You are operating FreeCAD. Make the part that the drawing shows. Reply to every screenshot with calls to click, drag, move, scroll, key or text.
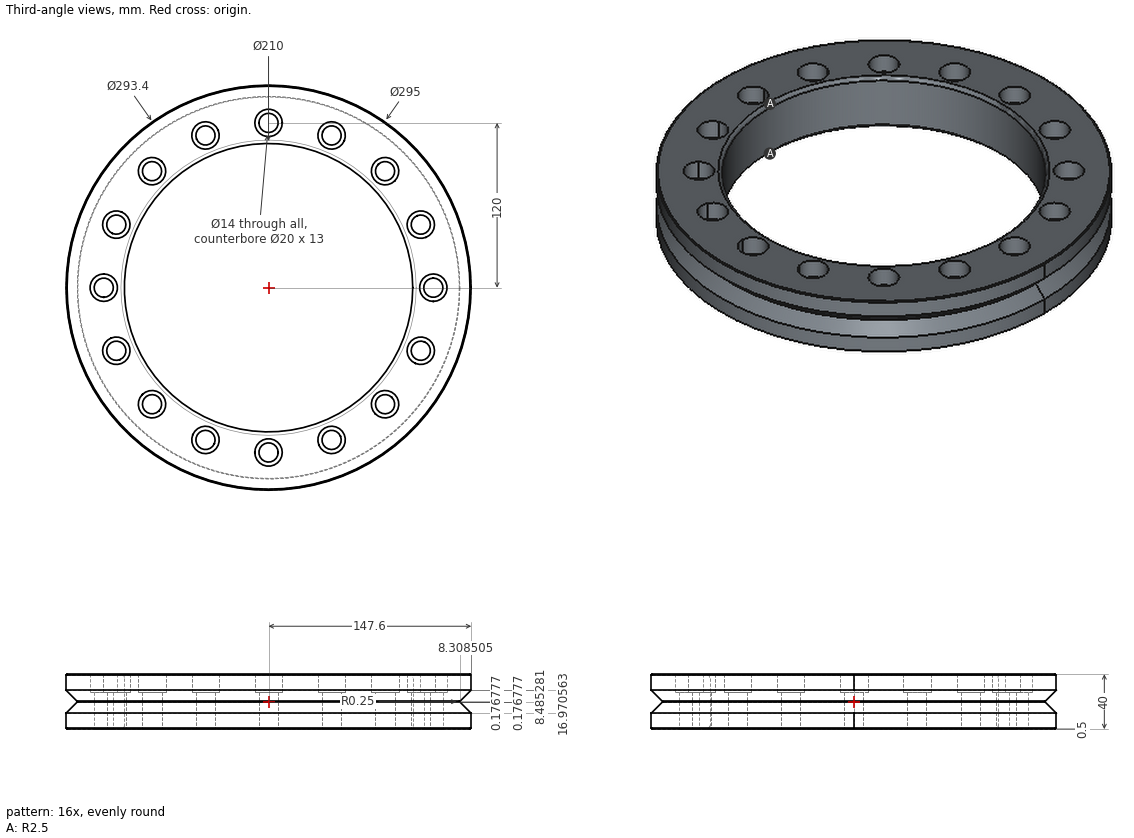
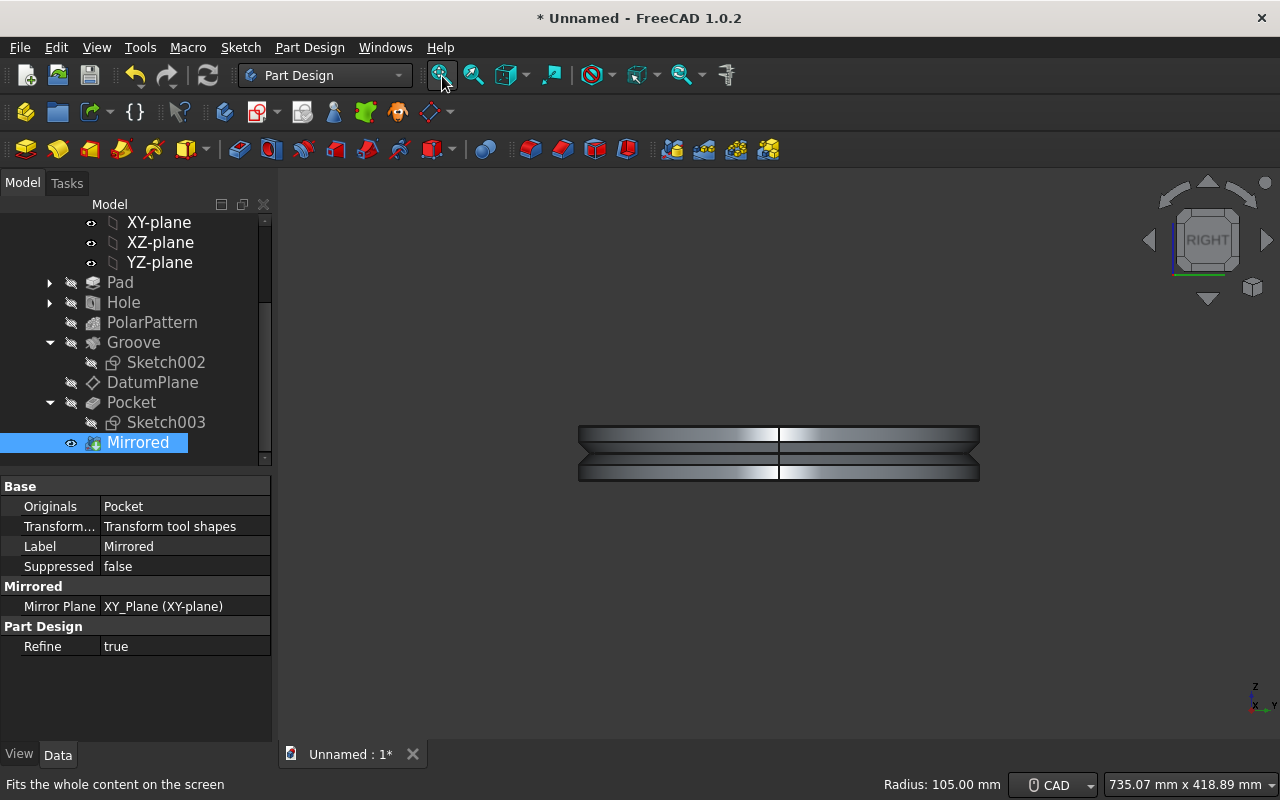
click(442, 76)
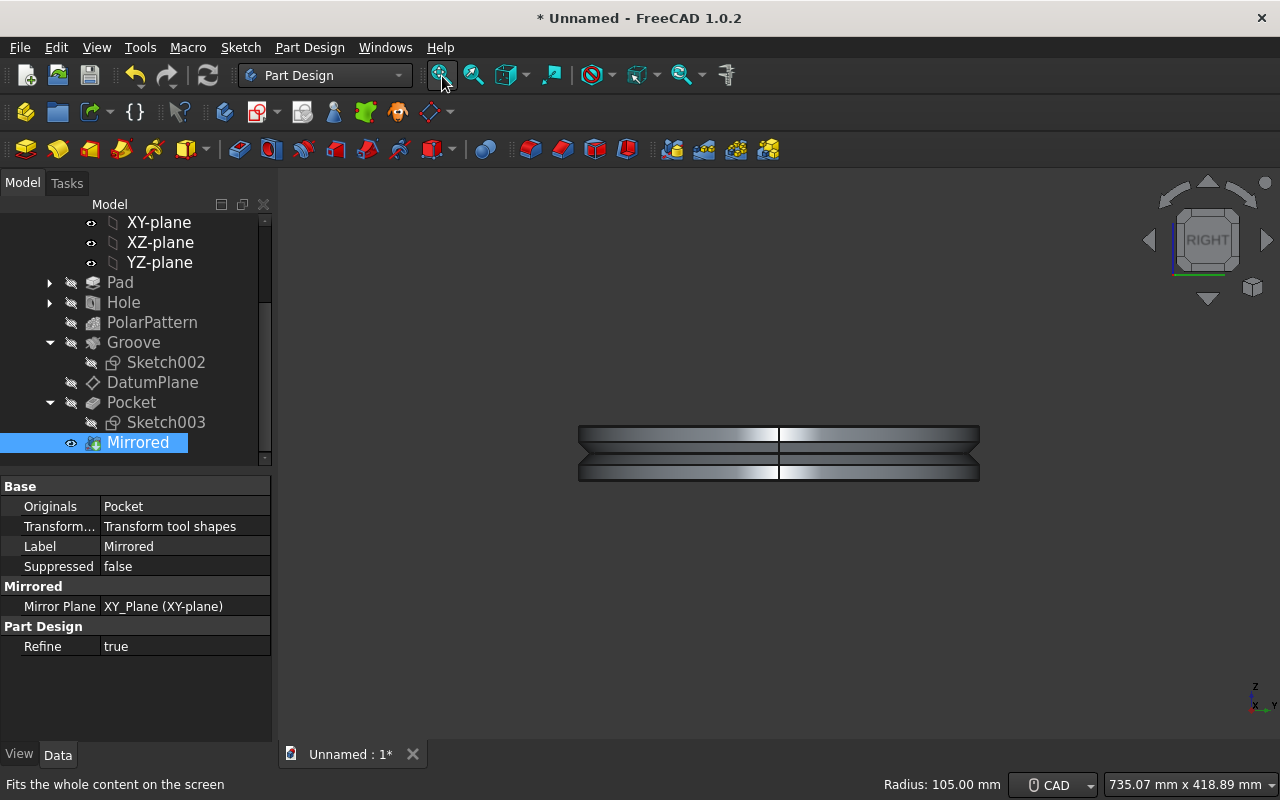
key(5)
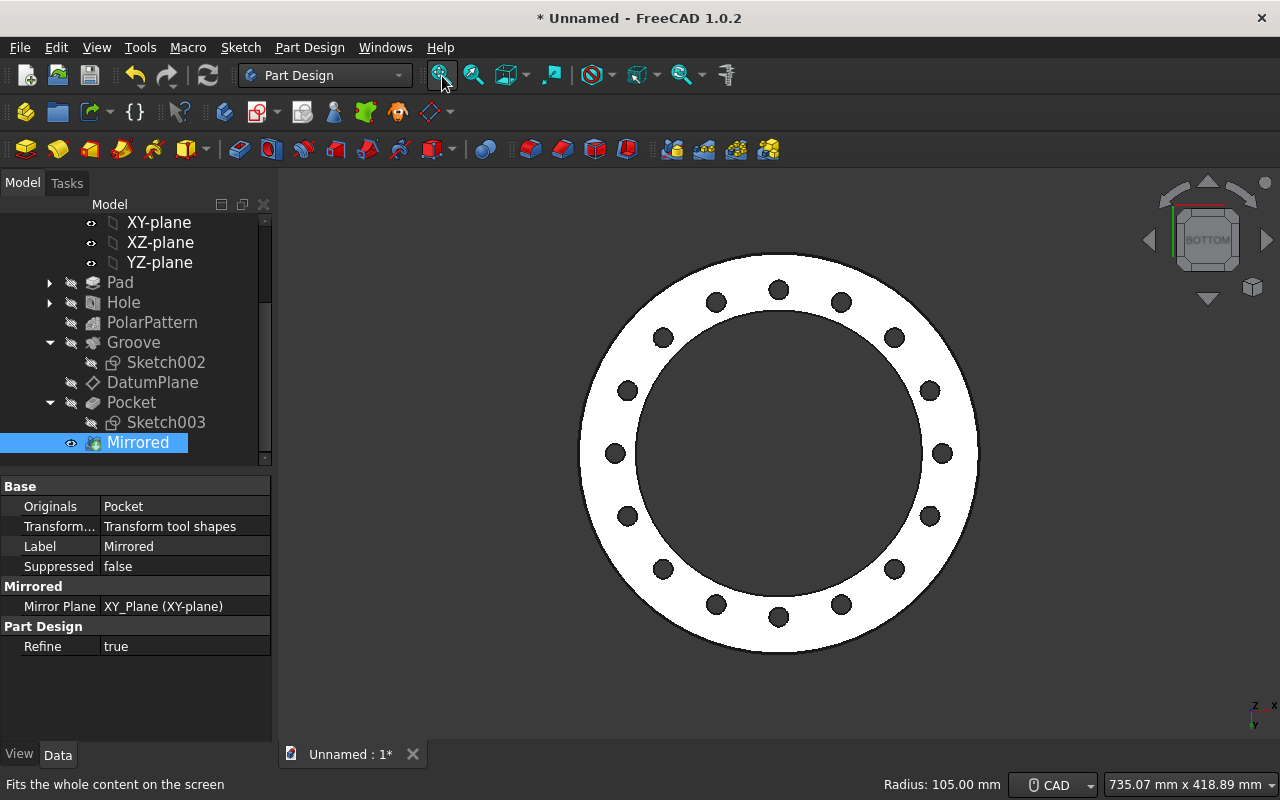
click(636, 452, ctrl)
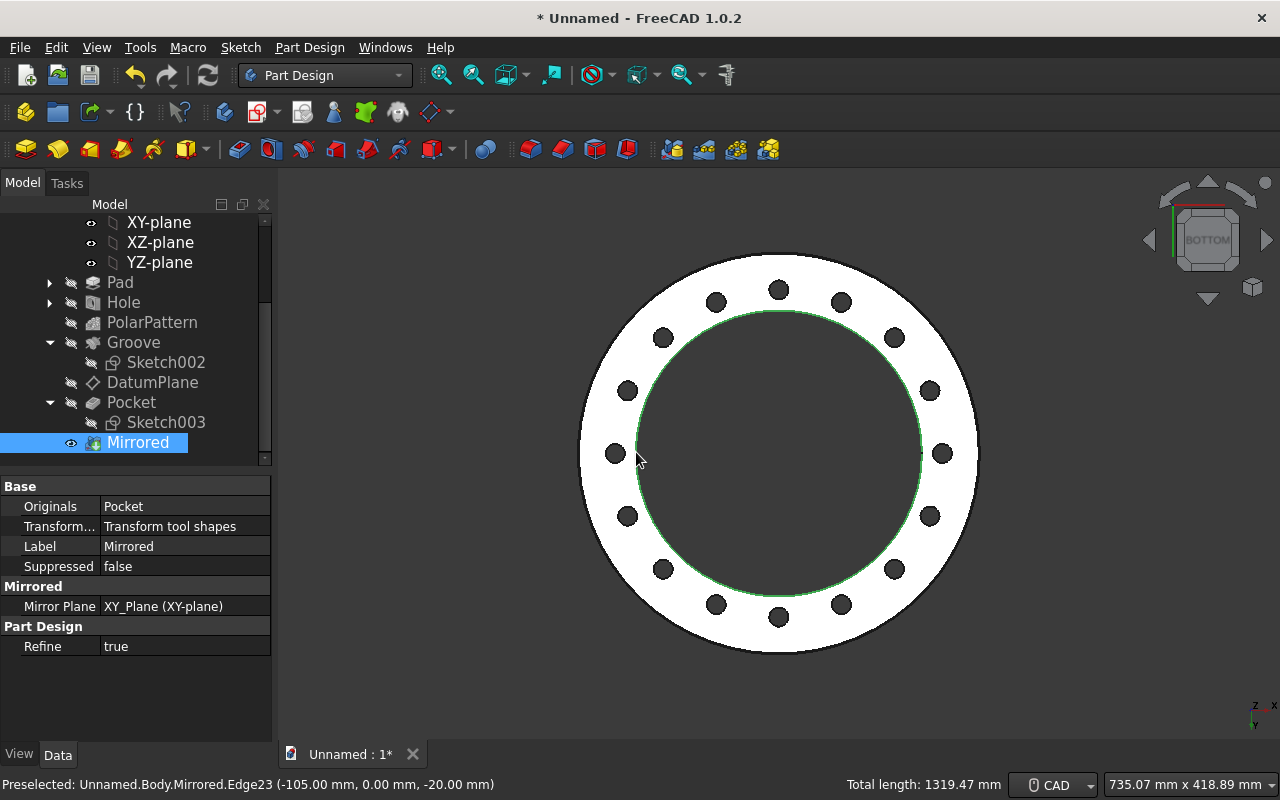
click(532, 150)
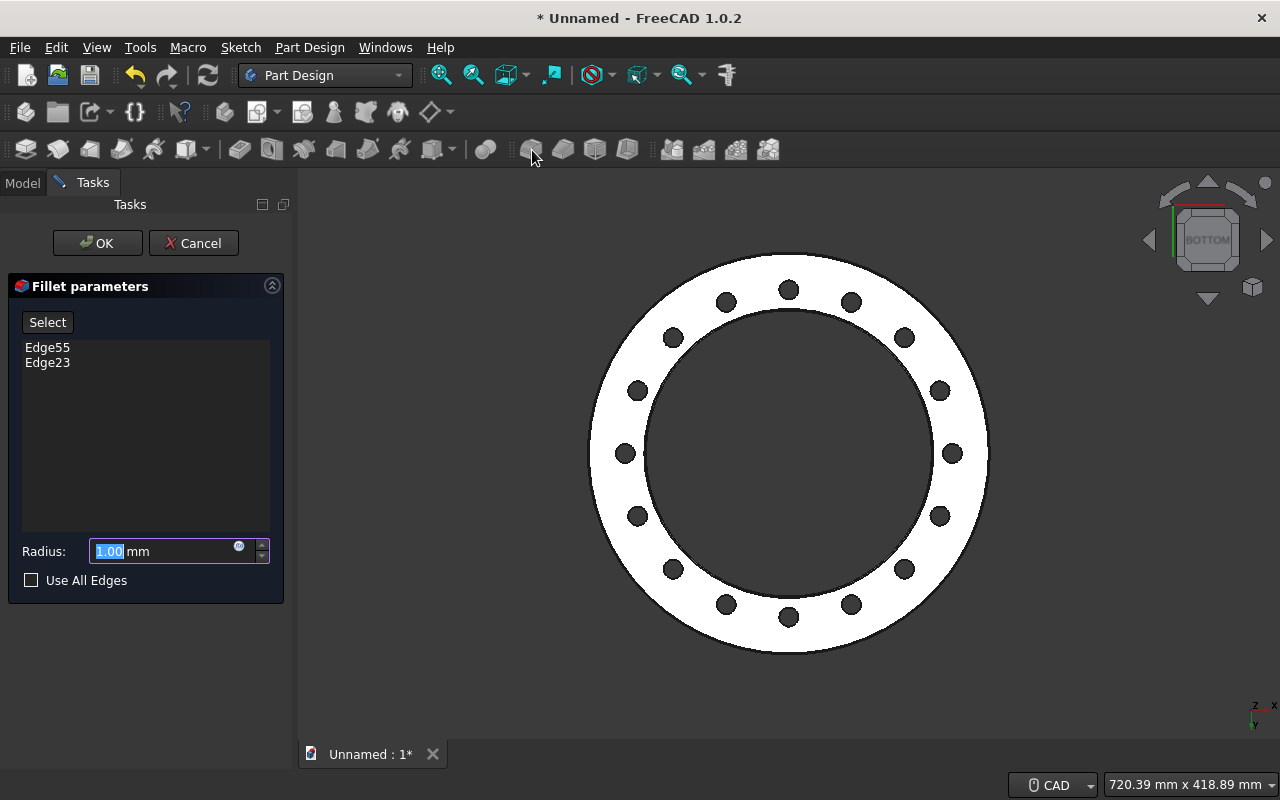
text(2.5)
key(Tab)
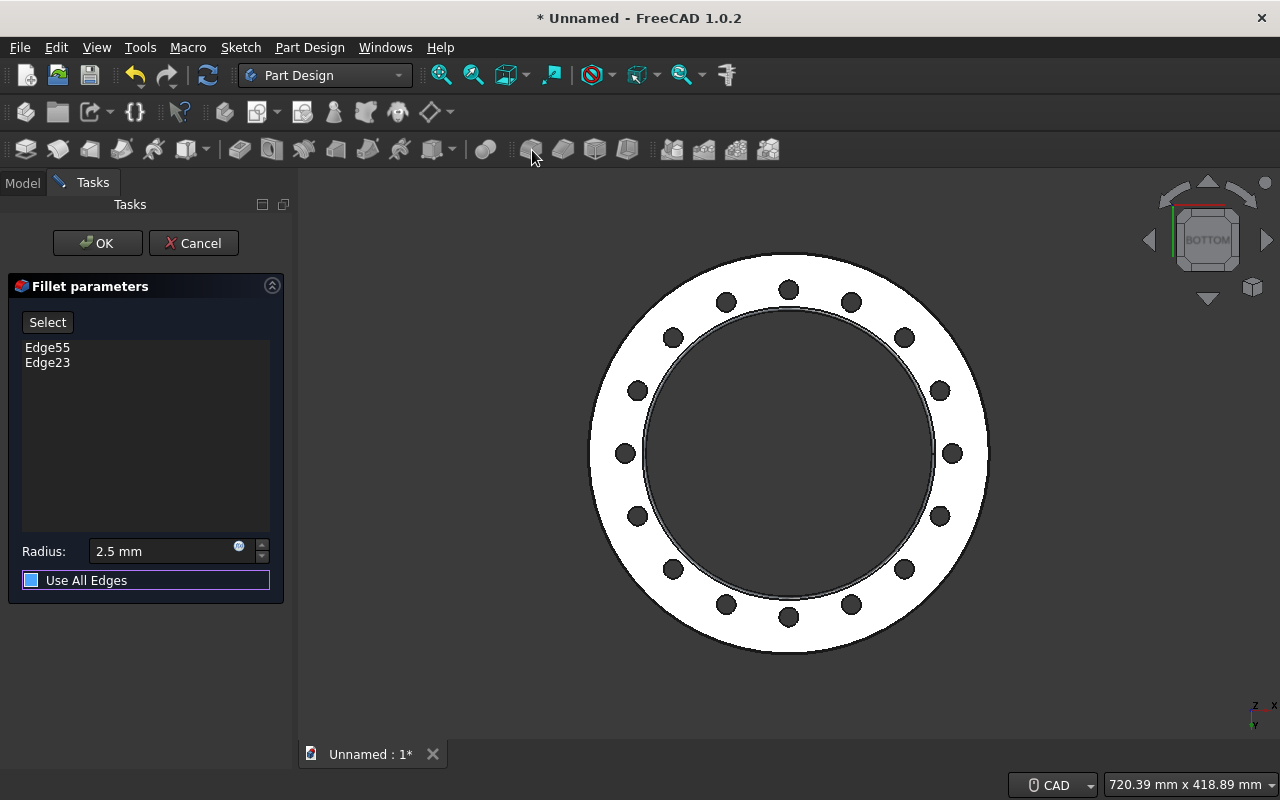
click(98, 243)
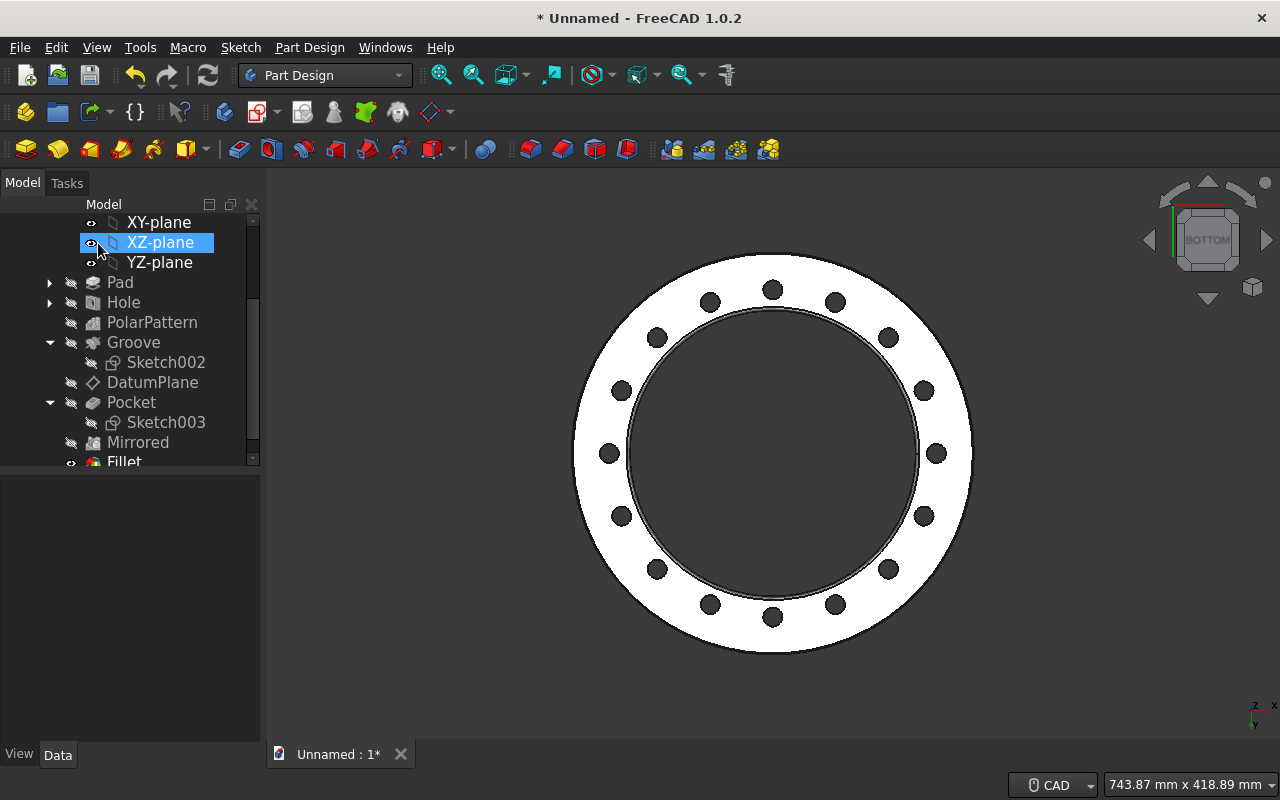
key(0)